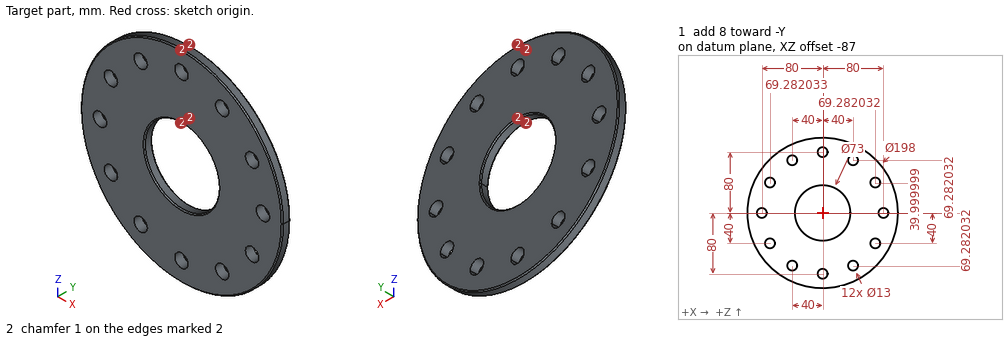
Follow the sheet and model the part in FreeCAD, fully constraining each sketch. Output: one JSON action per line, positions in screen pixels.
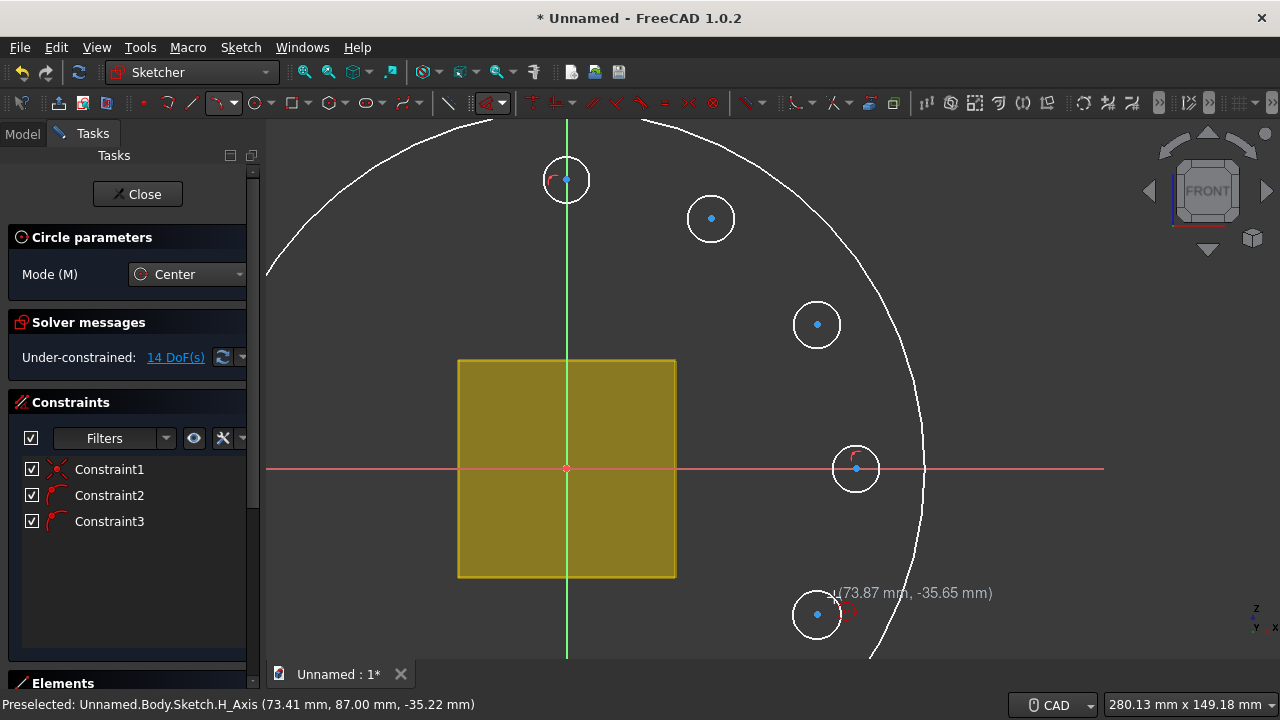
{"action": "scroll", "coordinate": [817, 324], "scroll_direction": "down", "scroll_amount": 4}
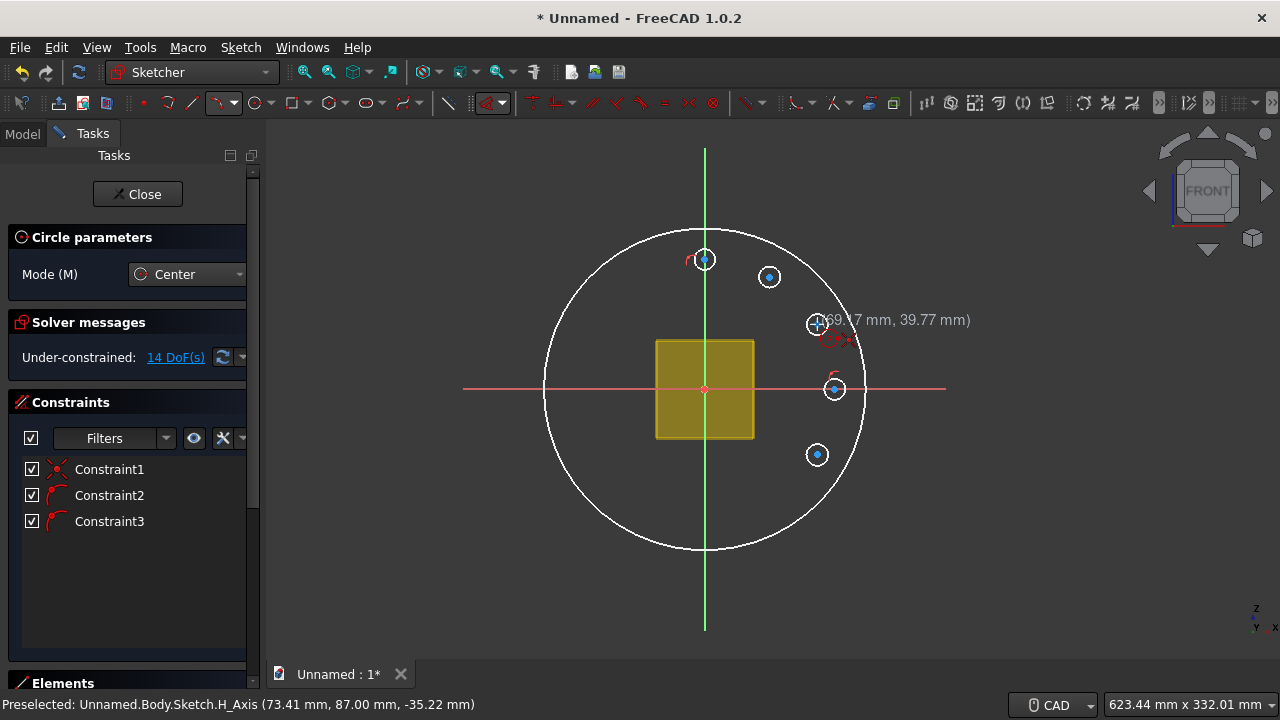
{"action": "scroll", "coordinate": [770, 502], "scroll_direction": "up", "scroll_amount": 4}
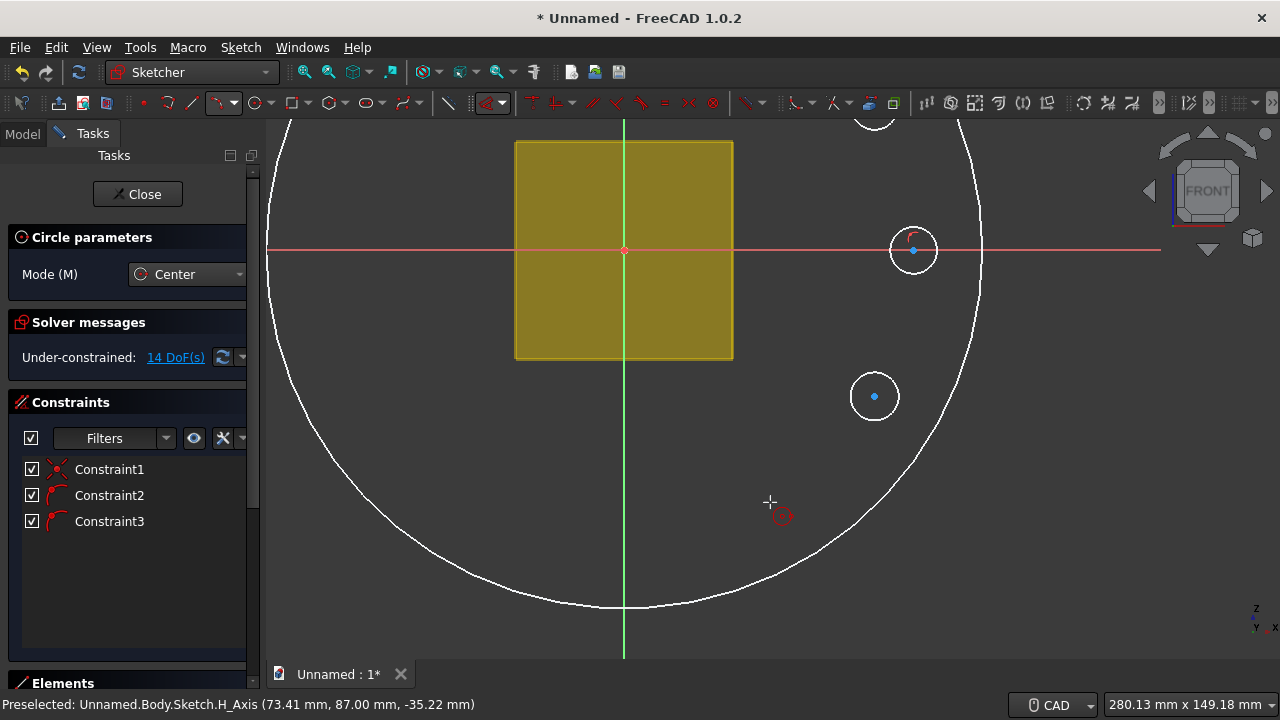
{"action": "left_click", "coordinate": [769, 501]}
{"action": "left_click", "coordinate": [786, 485]}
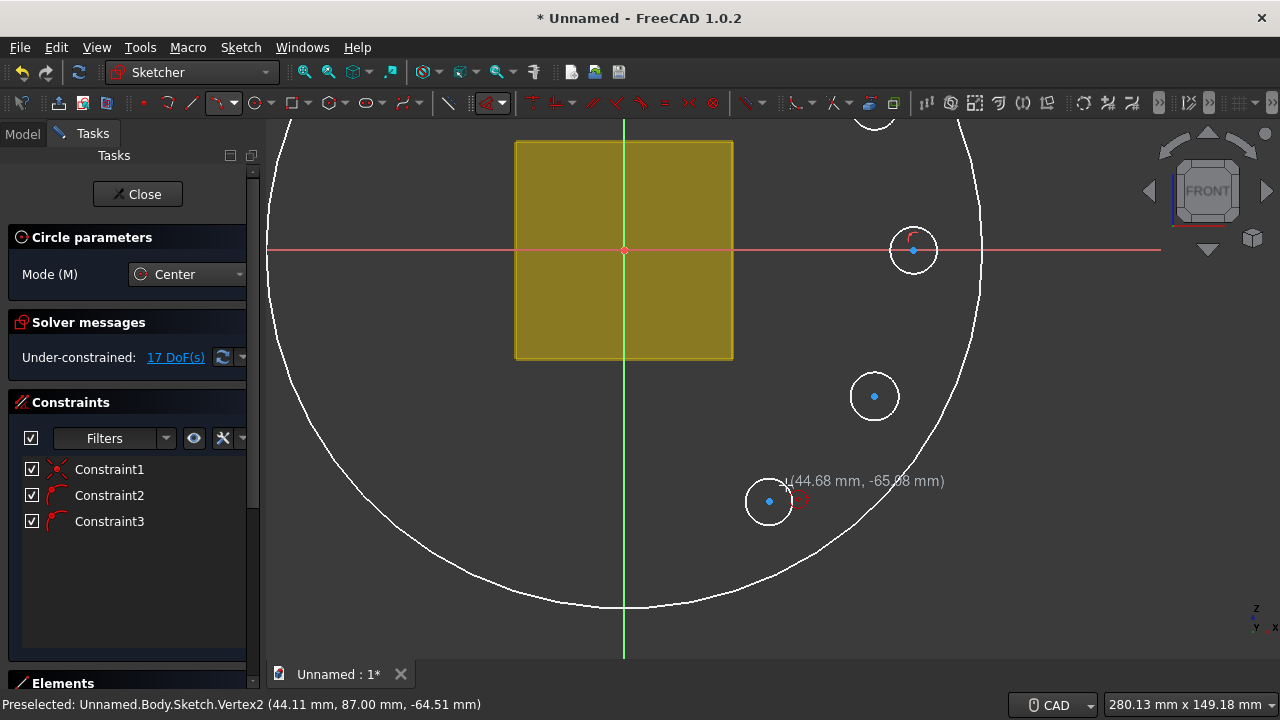
{"action": "scroll", "coordinate": [770, 502], "scroll_direction": "down", "scroll_amount": 4}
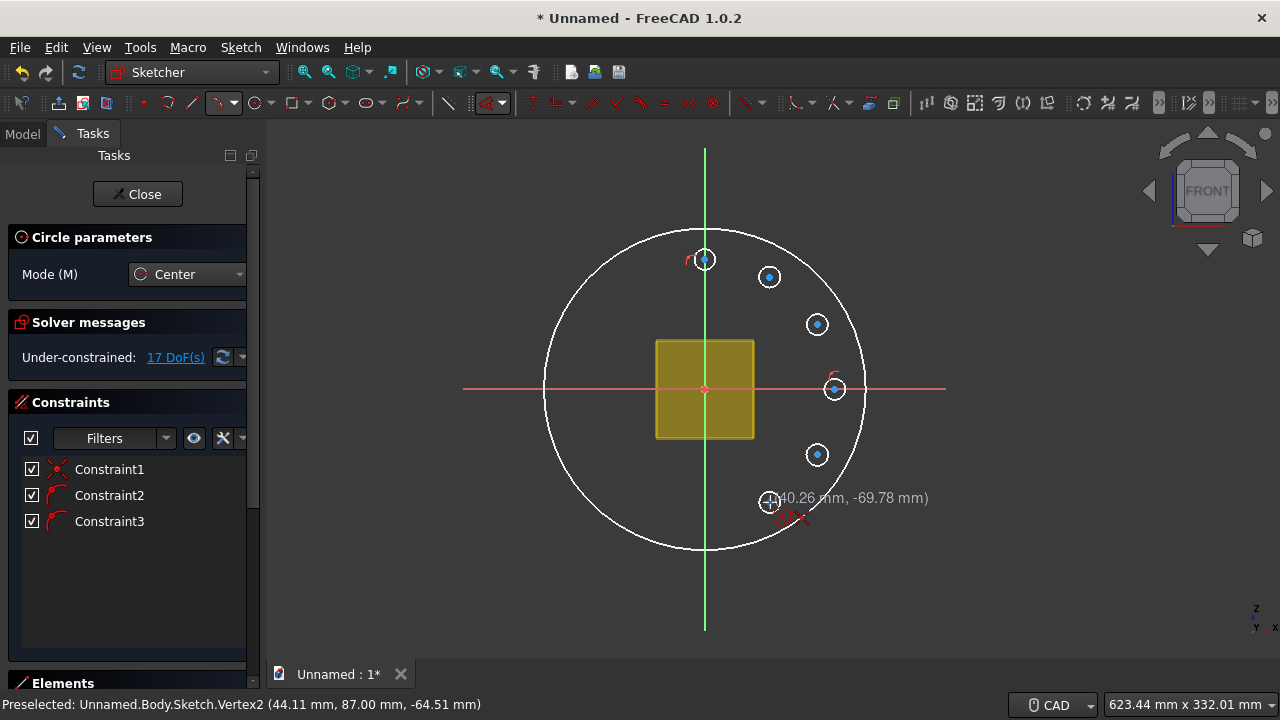
{"action": "scroll", "coordinate": [640, 277], "scroll_direction": "up", "scroll_amount": 4}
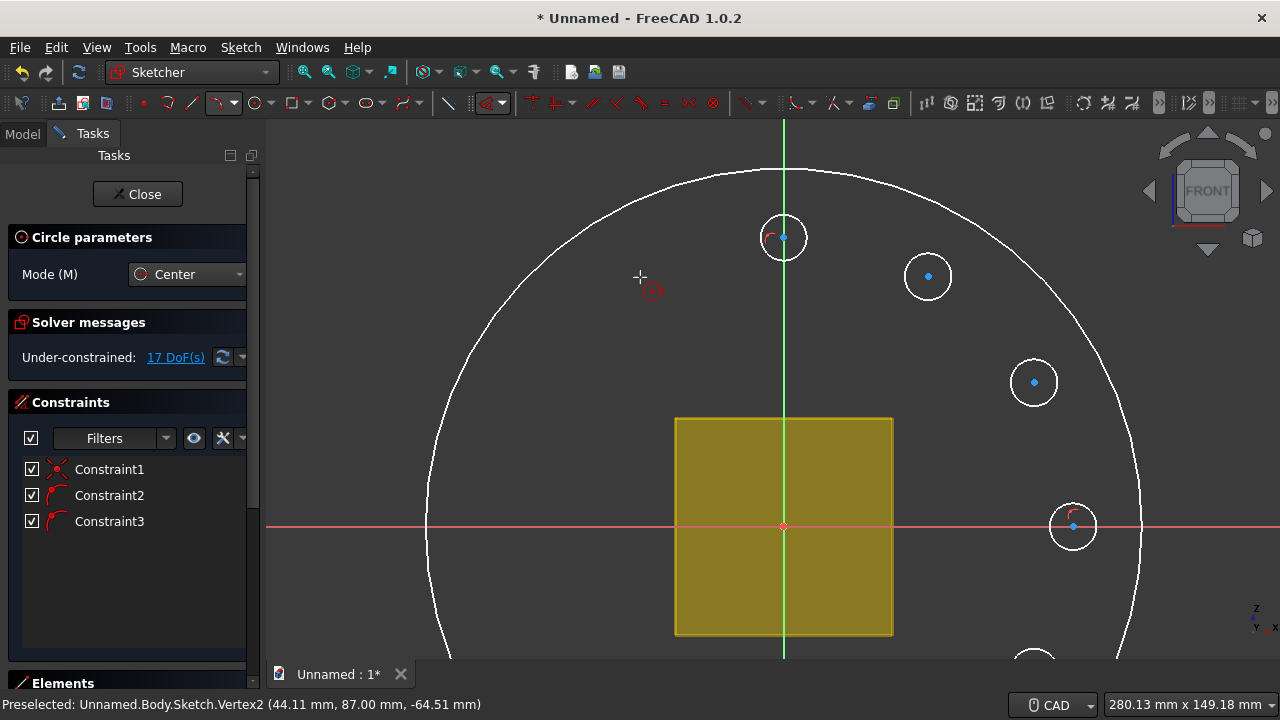
{"action": "left_click", "coordinate": [639, 276]}
{"action": "left_click", "coordinate": [656, 259]}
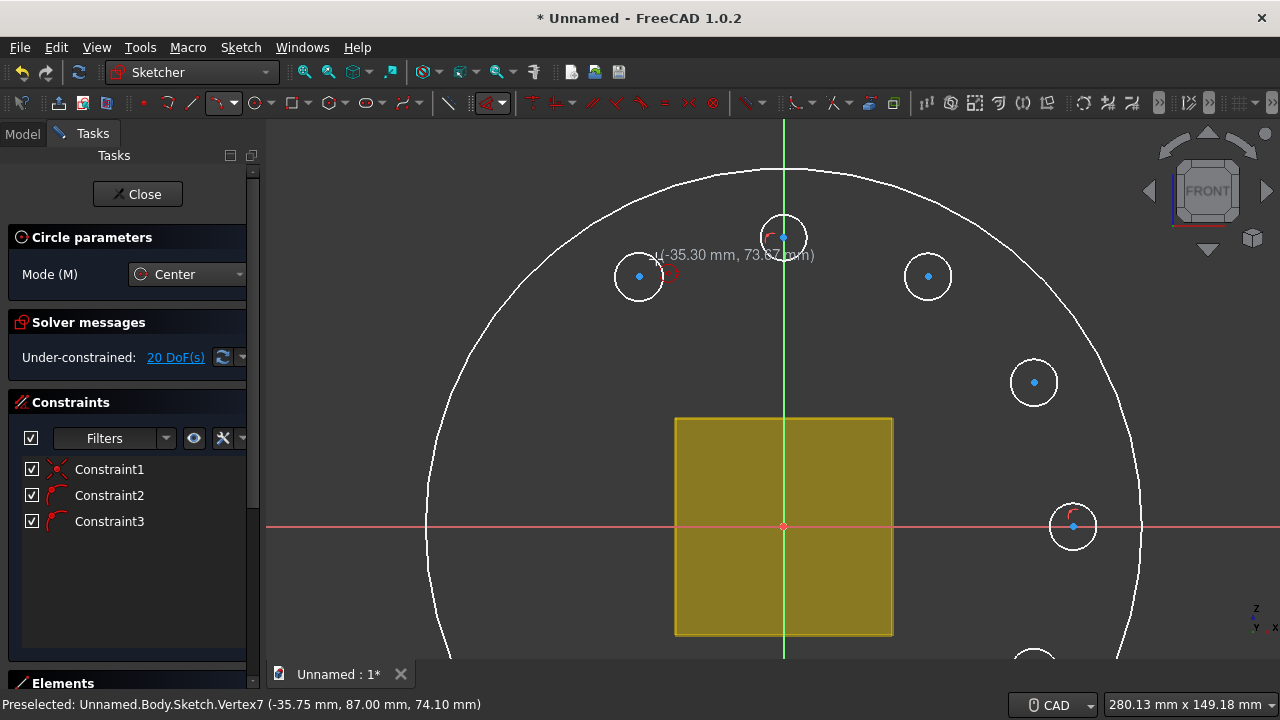
{"action": "left_click", "coordinate": [533, 382]}
{"action": "left_click", "coordinate": [550, 365]}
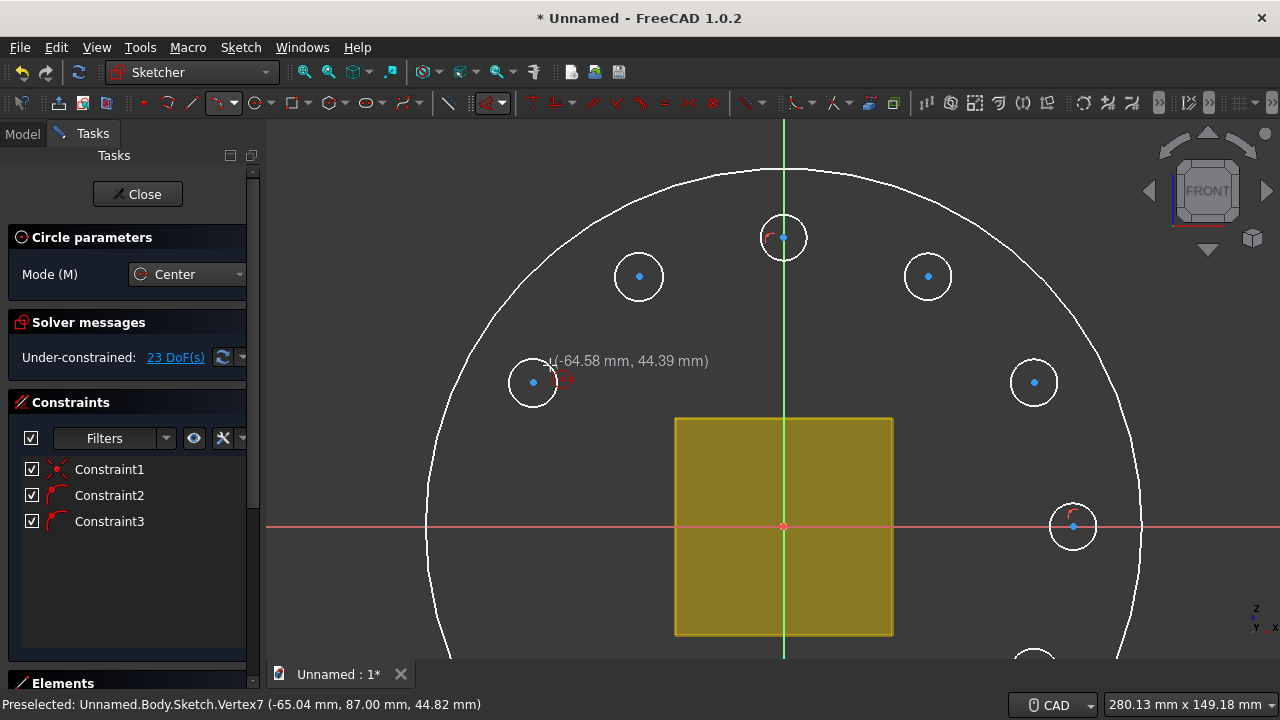
{"action": "left_click", "coordinate": [494, 527]}
{"action": "left_click", "coordinate": [511, 510]}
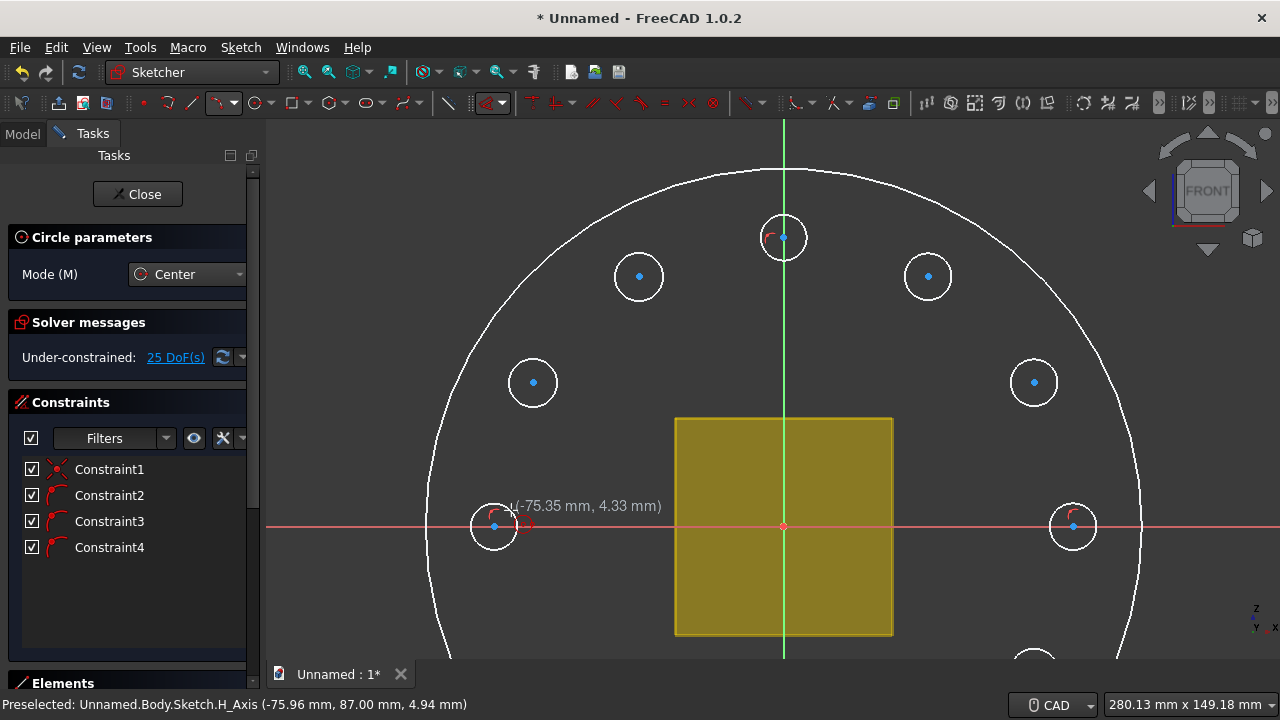
{"action": "left_click", "coordinate": [784, 527]}
{"action": "left_click", "coordinate": [877, 433]}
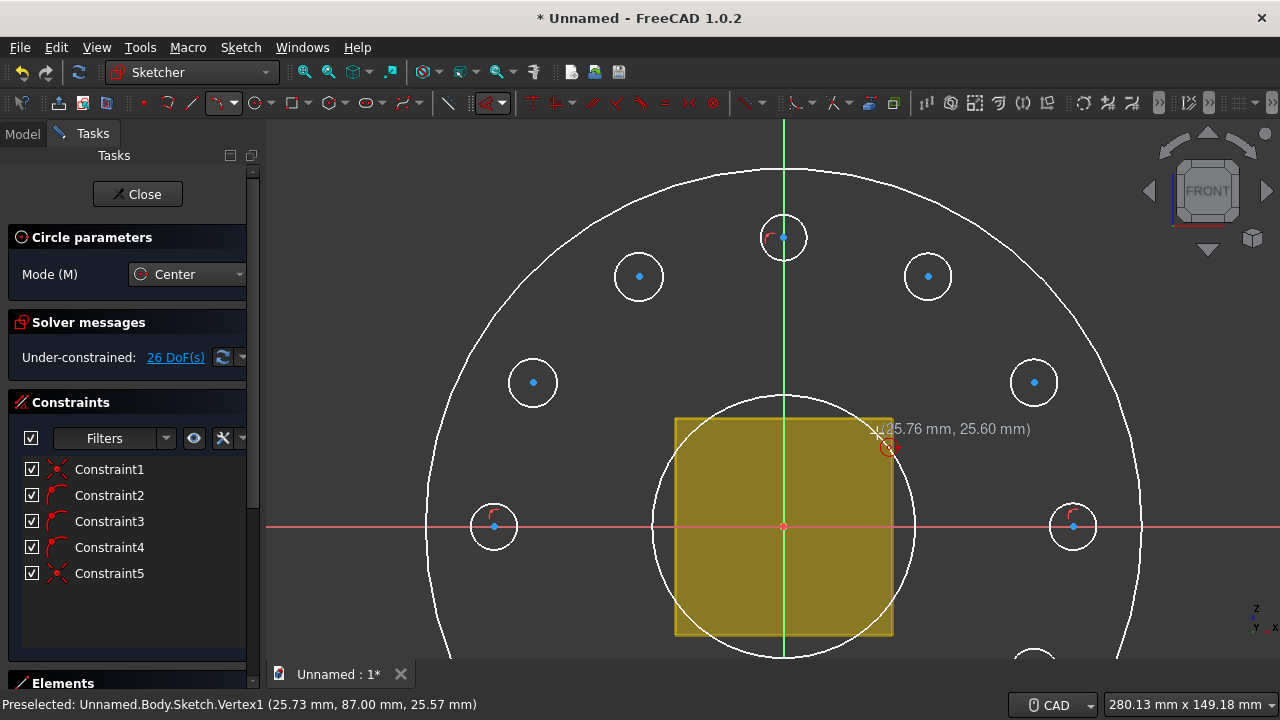
{"action": "scroll", "coordinate": [640, 277], "scroll_direction": "down", "scroll_amount": 4}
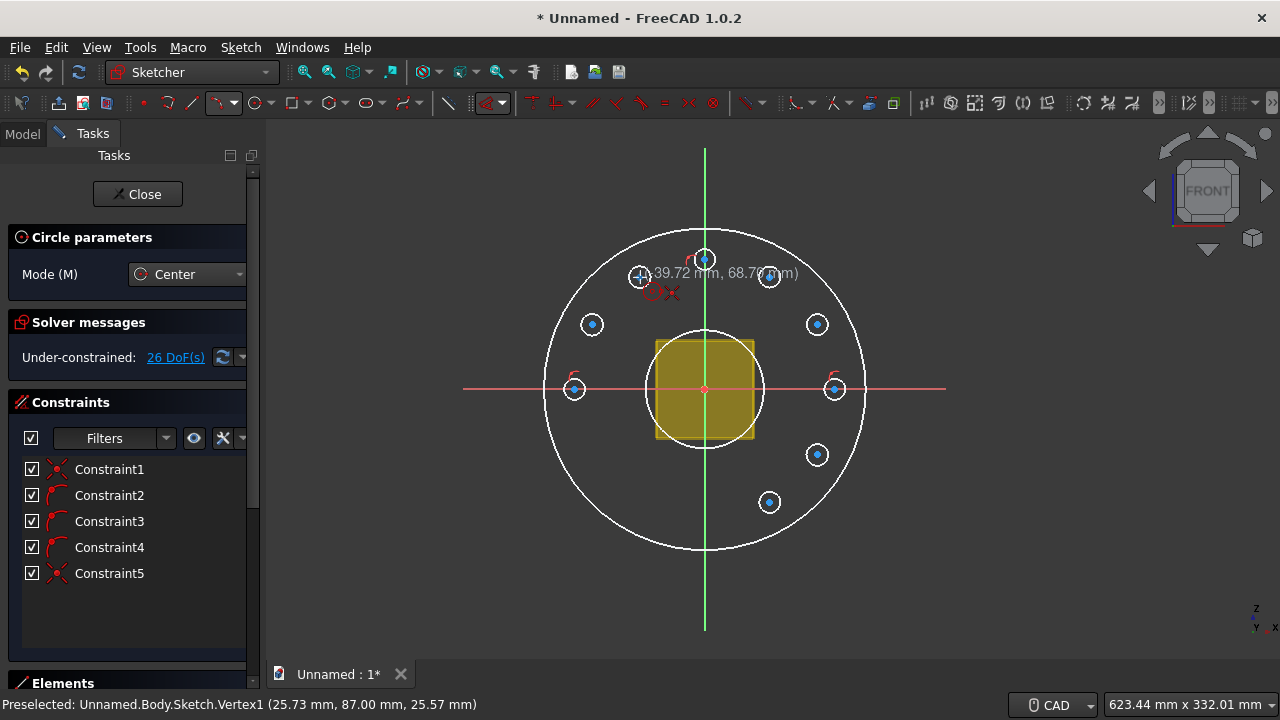
{"action": "scroll", "coordinate": [705, 519], "scroll_direction": "up", "scroll_amount": 4}